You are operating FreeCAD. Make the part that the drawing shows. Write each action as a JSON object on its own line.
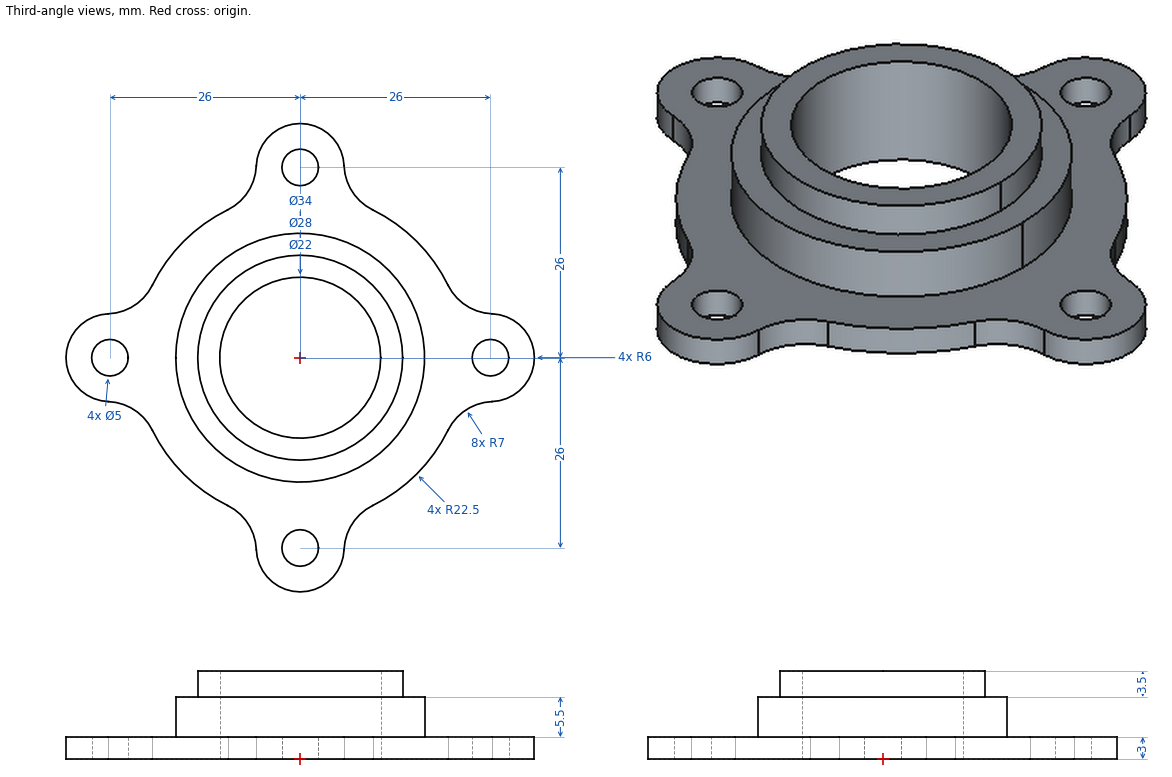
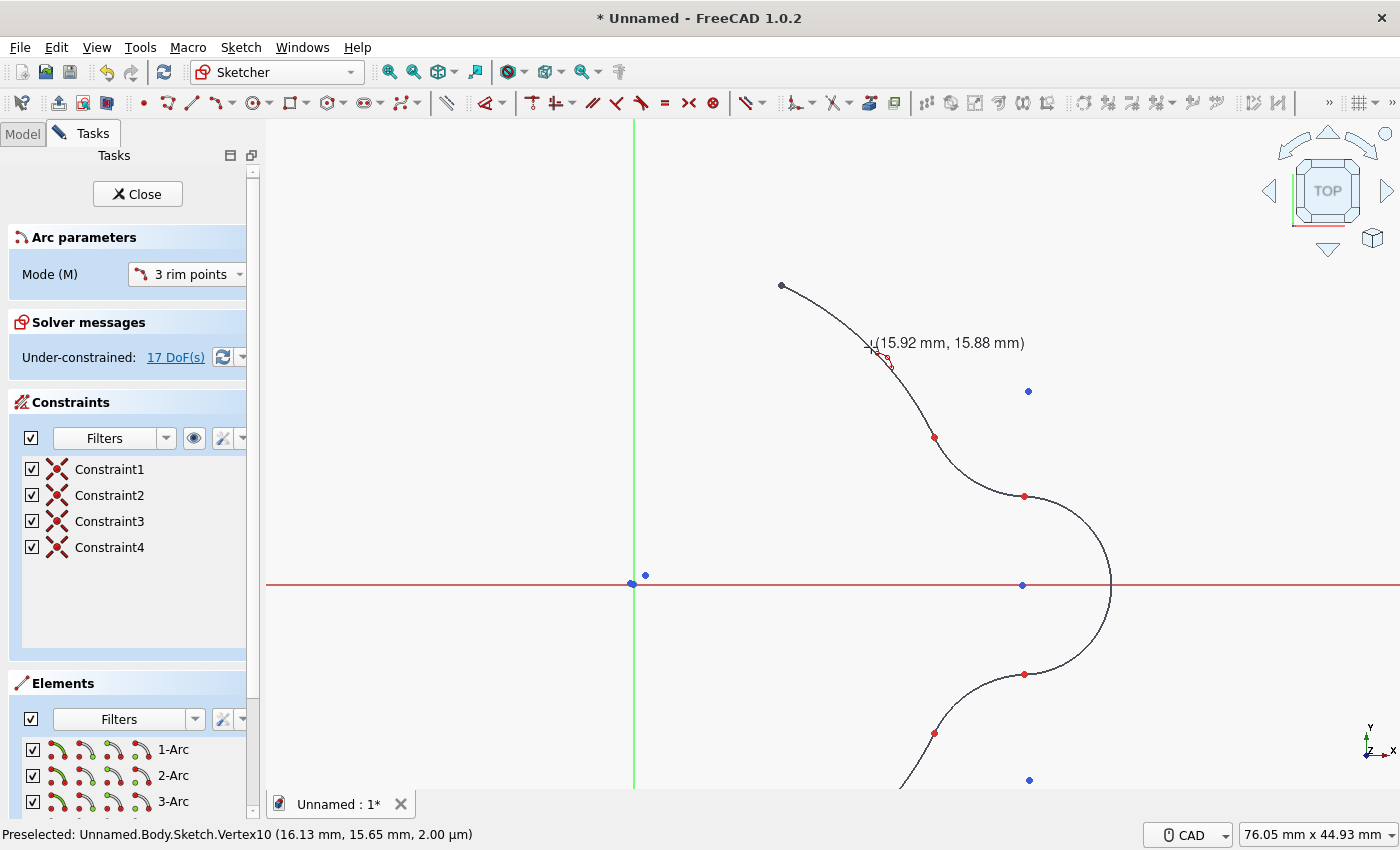
{"action": "left_click", "coordinate": [781, 285]}
{"action": "left_click", "coordinate": [723, 194]}
{"action": "left_click", "coordinate": [740, 247]}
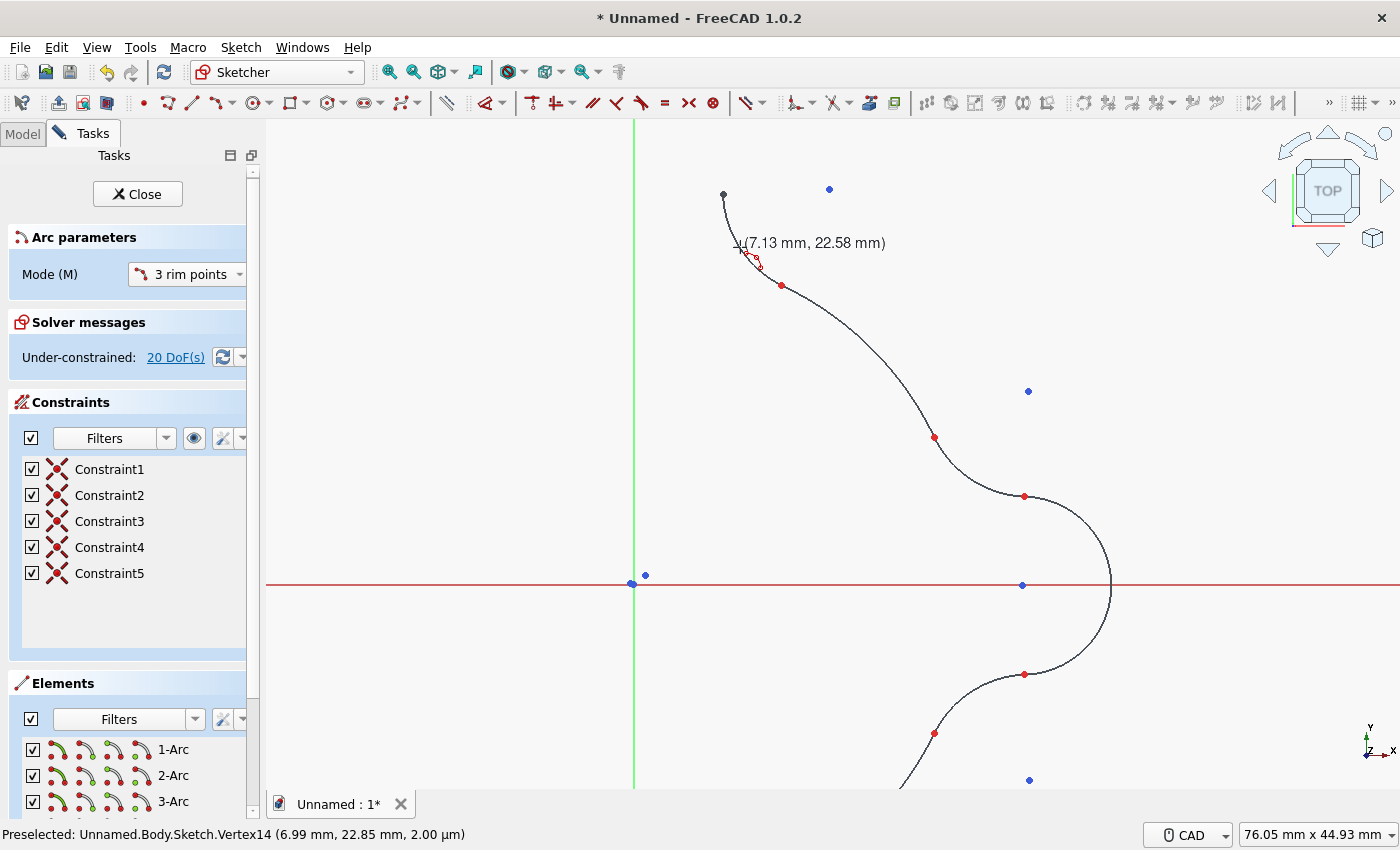
{"action": "left_click", "coordinate": [723, 195]}
{"action": "left_click", "coordinate": [544, 194]}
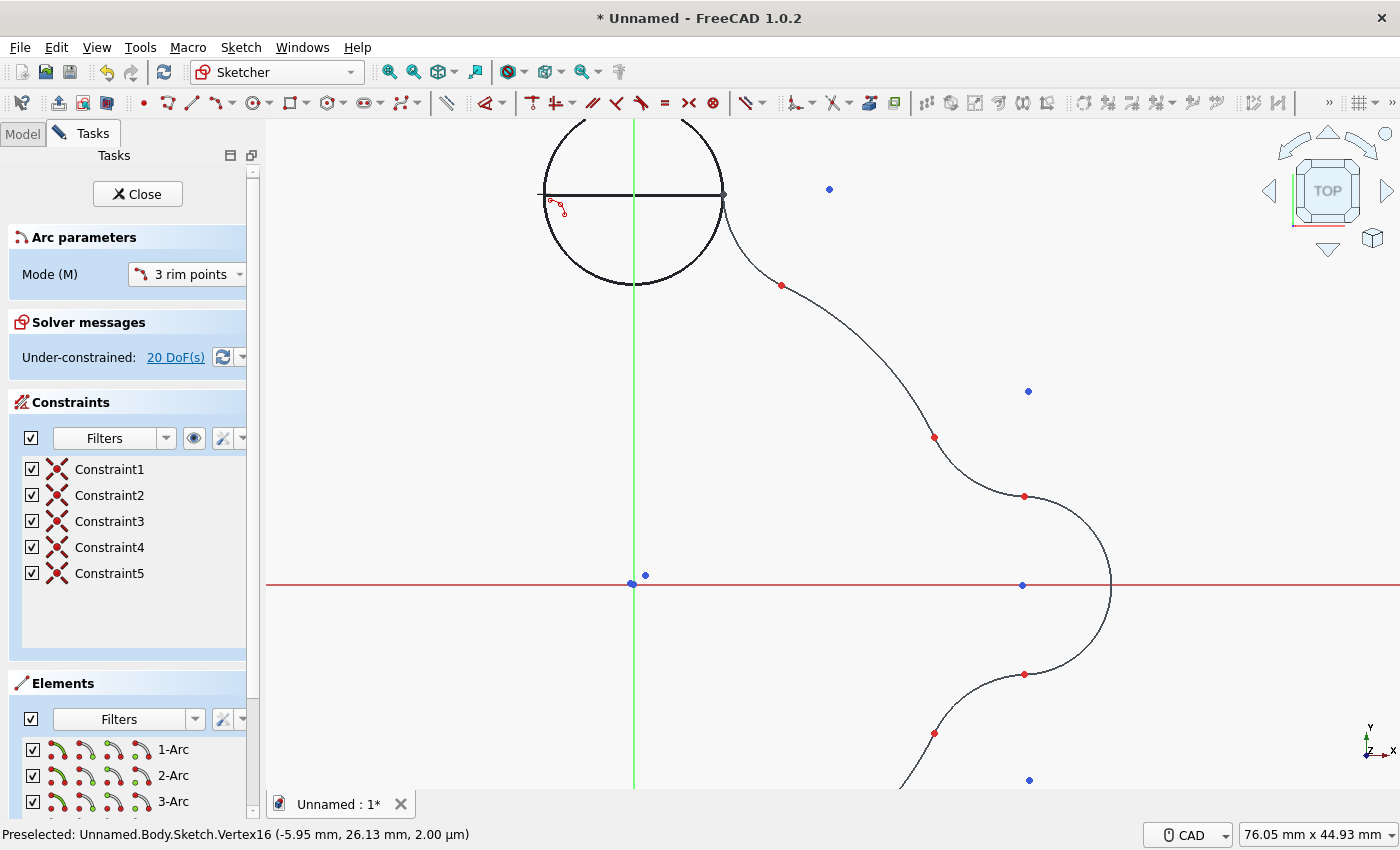
{"action": "scroll", "coordinate": [871, 347], "scroll_direction": "down", "scroll_amount": 4}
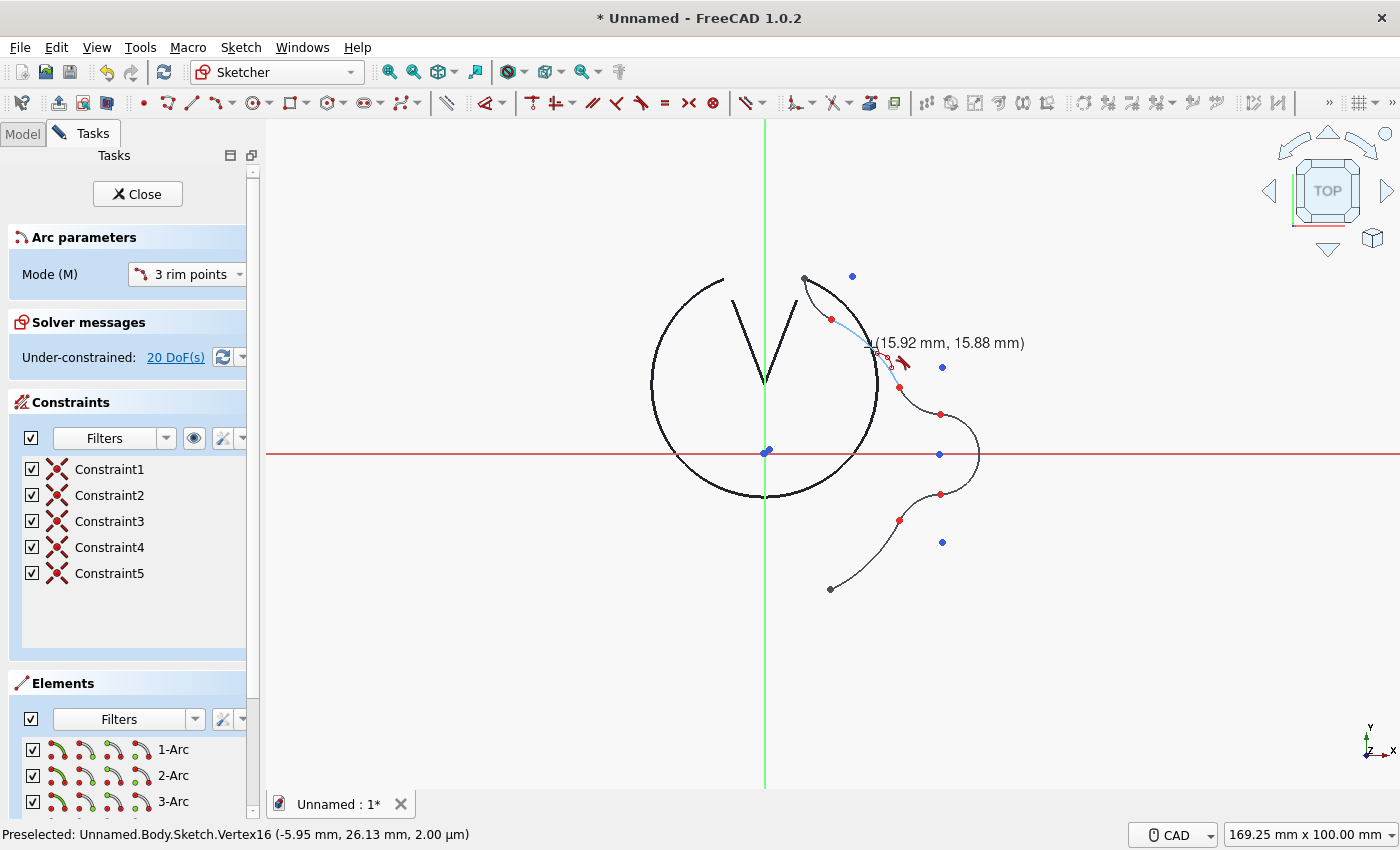
{"action": "left_click", "coordinate": [788, 247]}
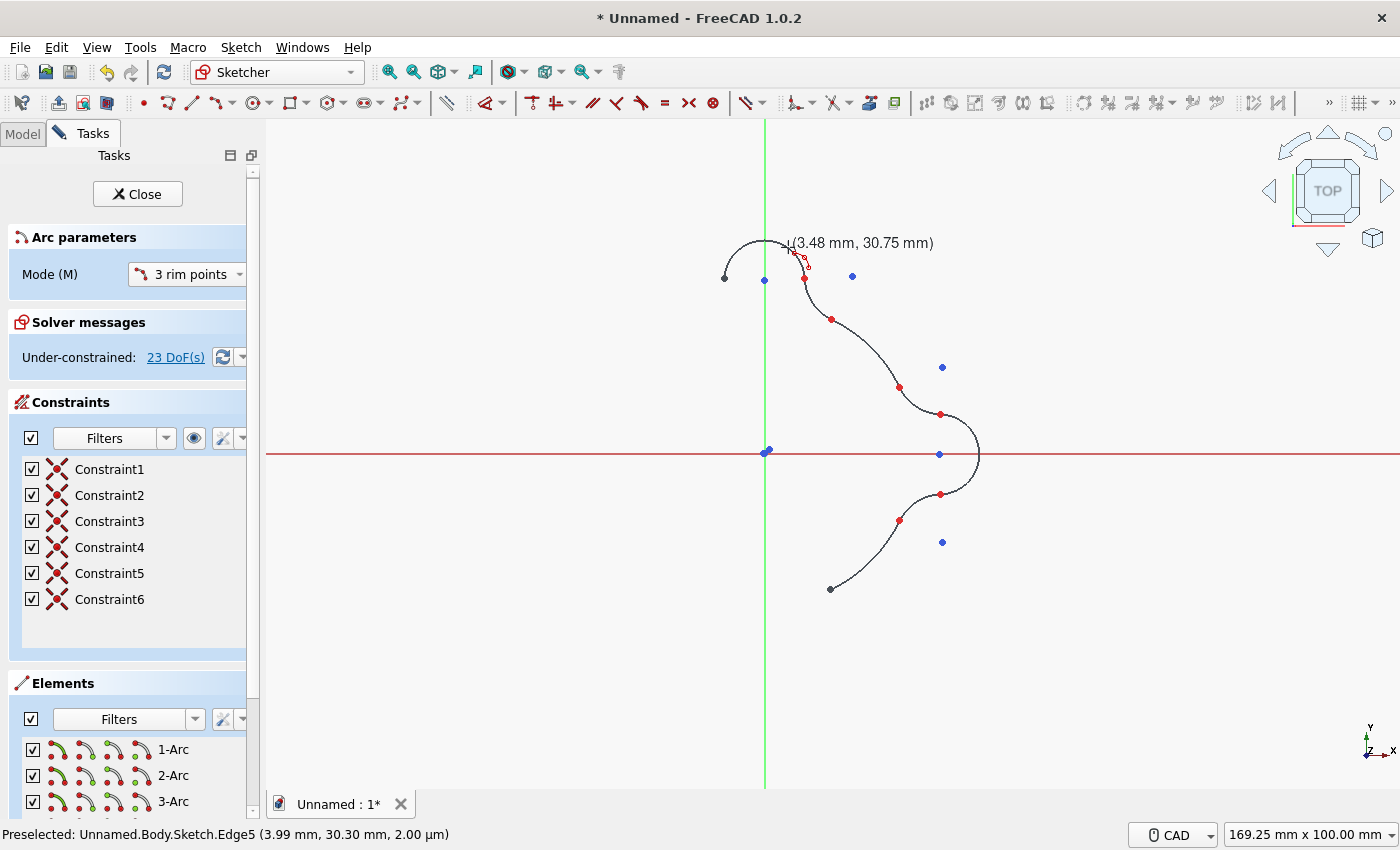
{"action": "left_click", "coordinate": [724, 279]}
{"action": "left_click", "coordinate": [698, 319]}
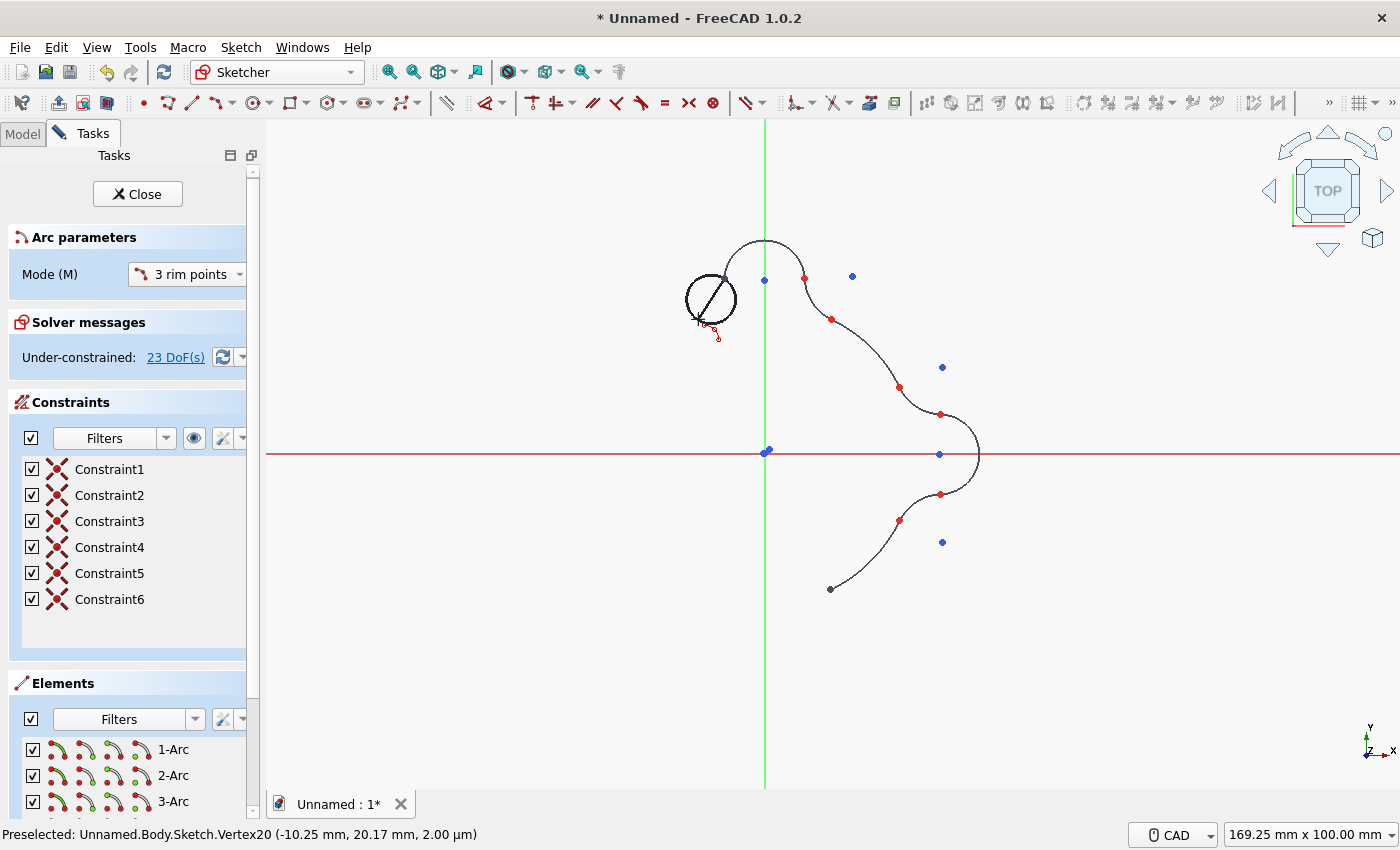
{"action": "scroll", "coordinate": [717, 302], "scroll_direction": "up", "scroll_amount": 5}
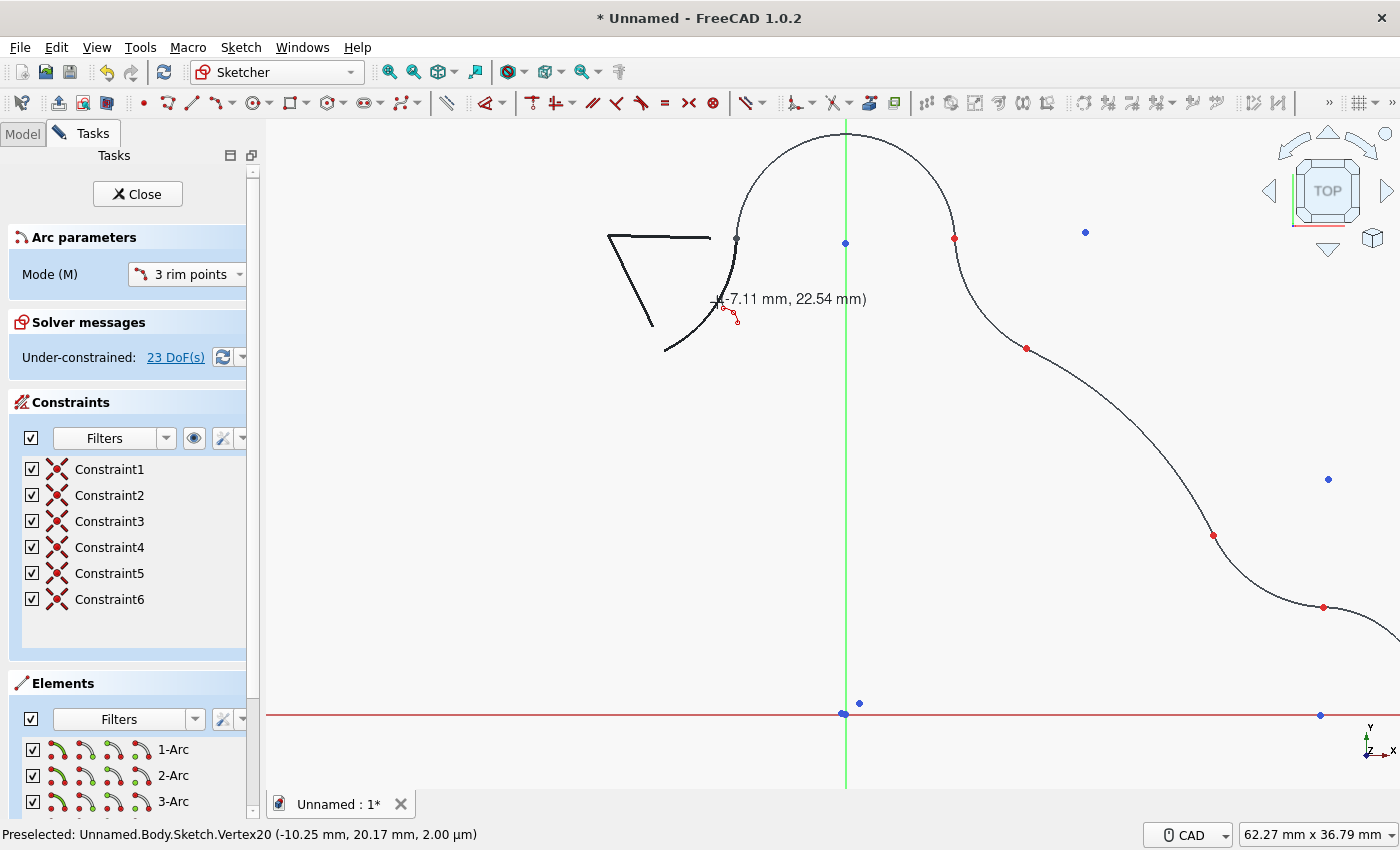
{"action": "left_click", "coordinate": [716, 302]}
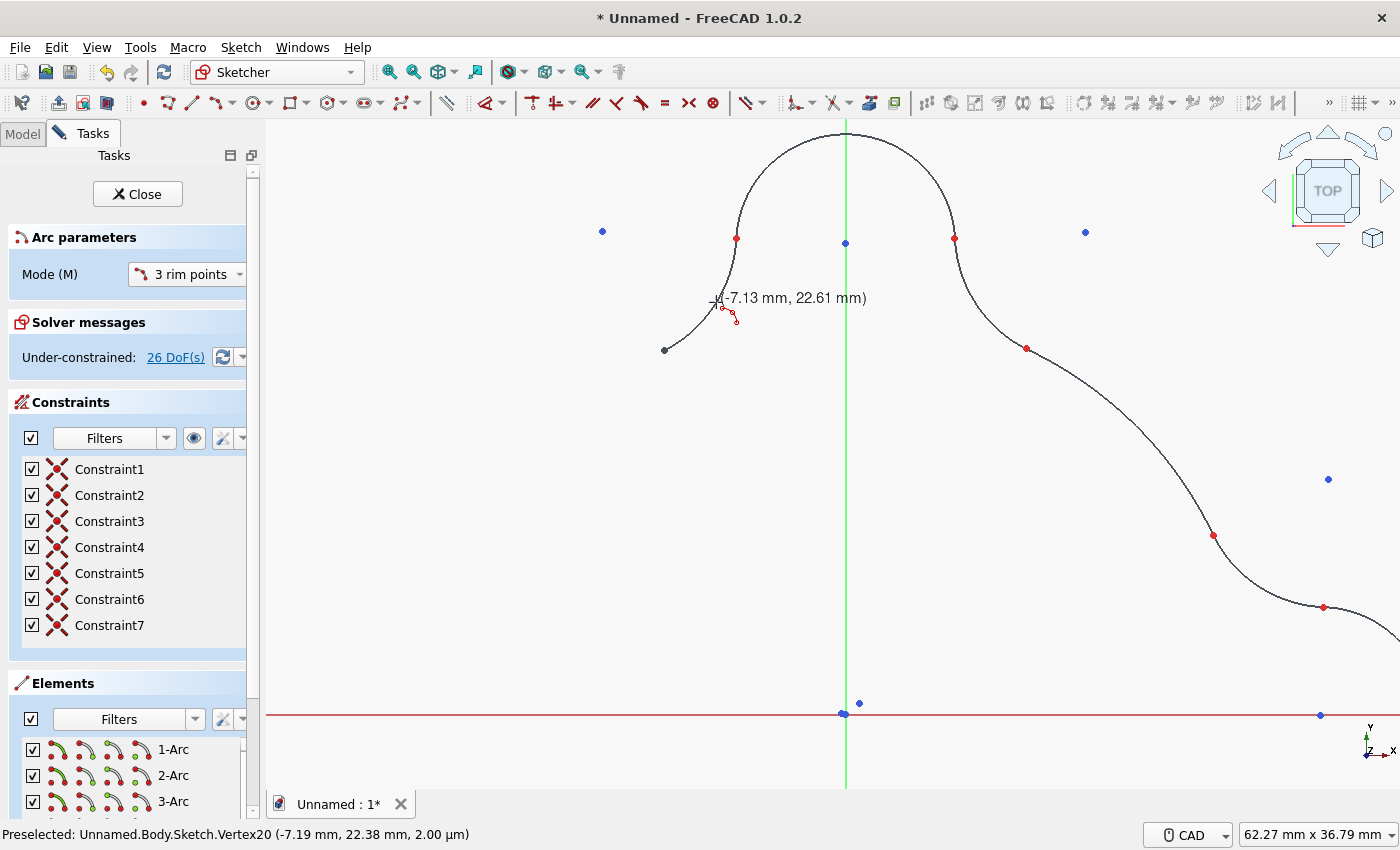
{"action": "left_click", "coordinate": [665, 350]}
{"action": "left_click", "coordinate": [478, 534]}
{"action": "left_click", "coordinate": [556, 425]}